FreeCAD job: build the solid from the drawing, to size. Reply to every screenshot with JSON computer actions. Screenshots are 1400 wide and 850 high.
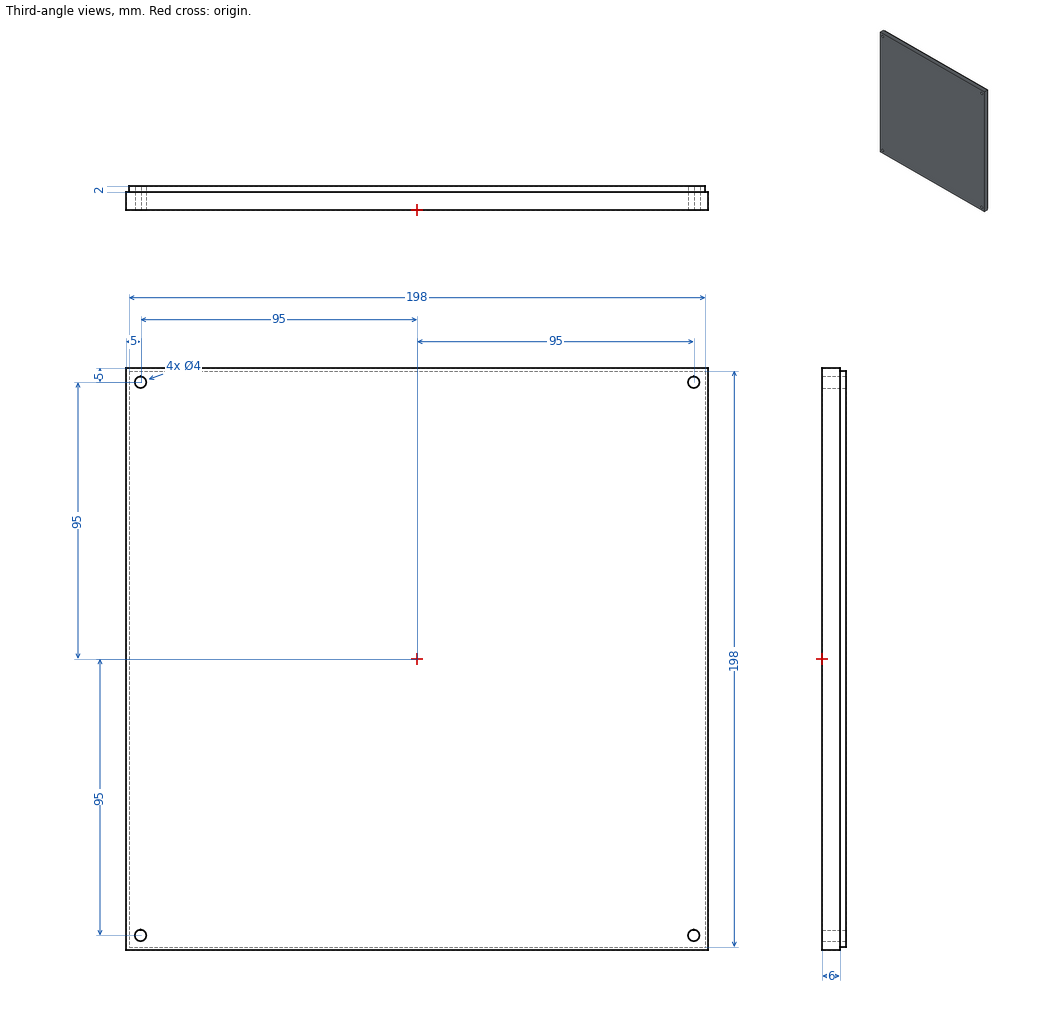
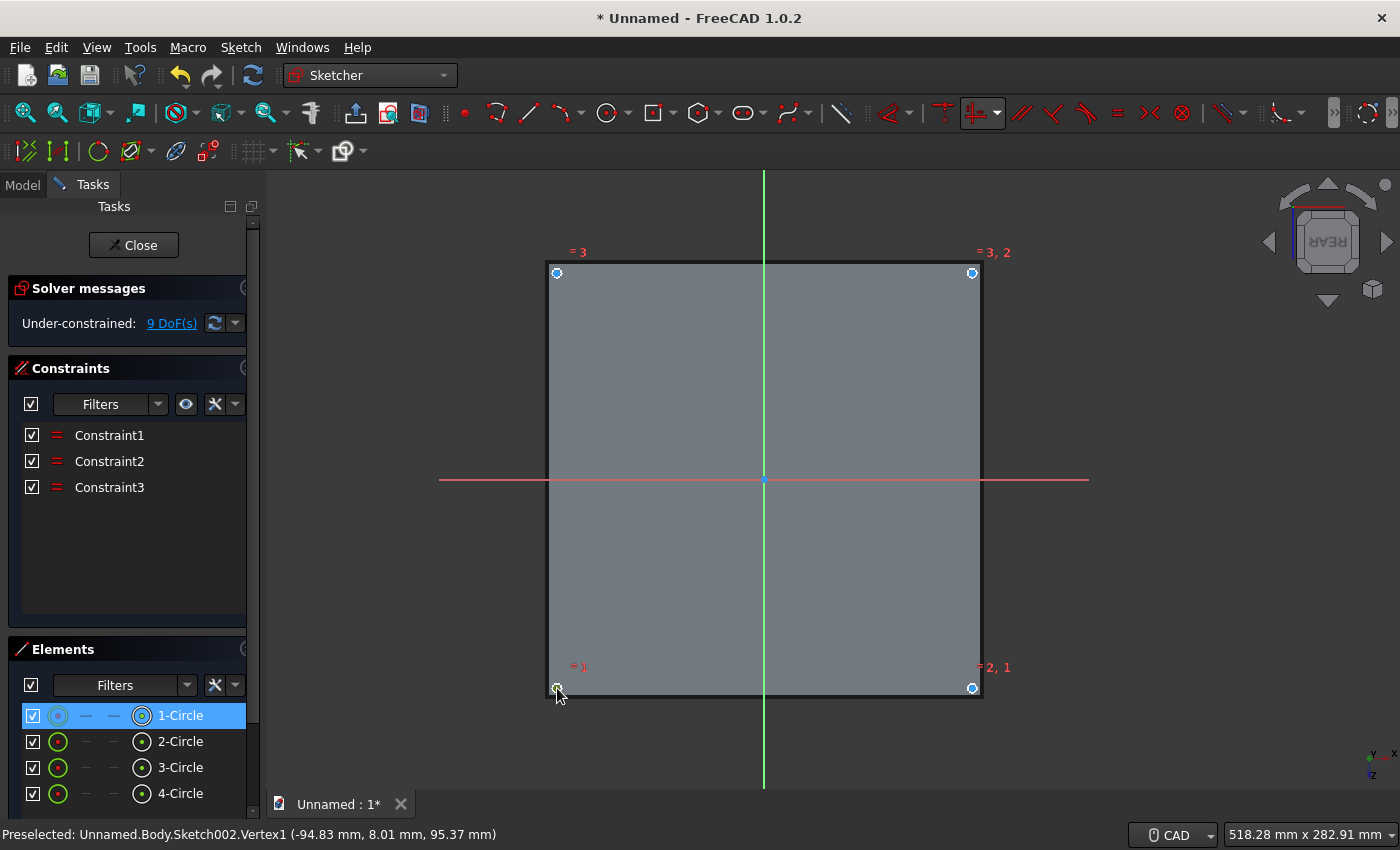
{"action": "left_click", "coordinate": [972, 688]}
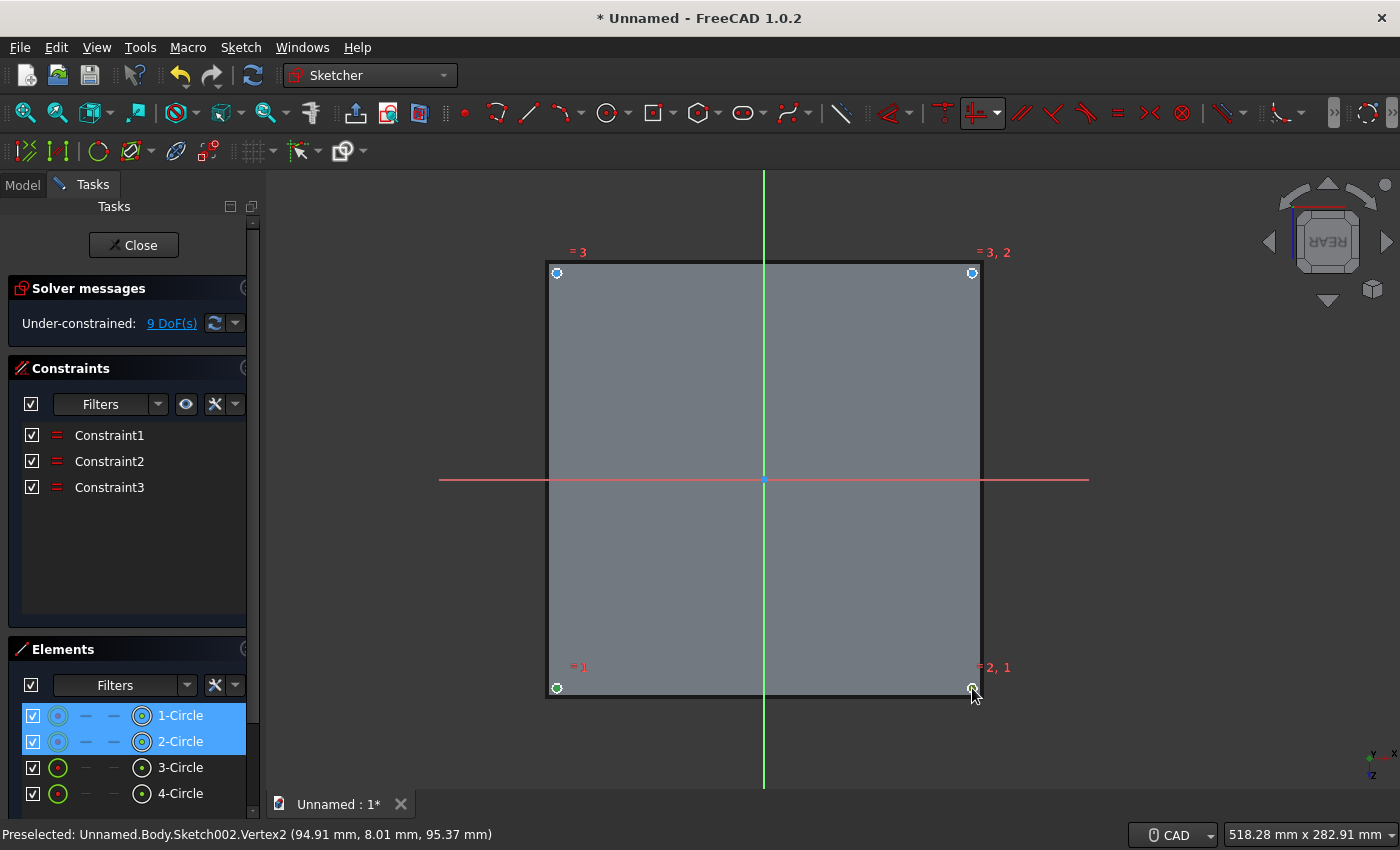
{"action": "left_click", "coordinate": [1000, 114]}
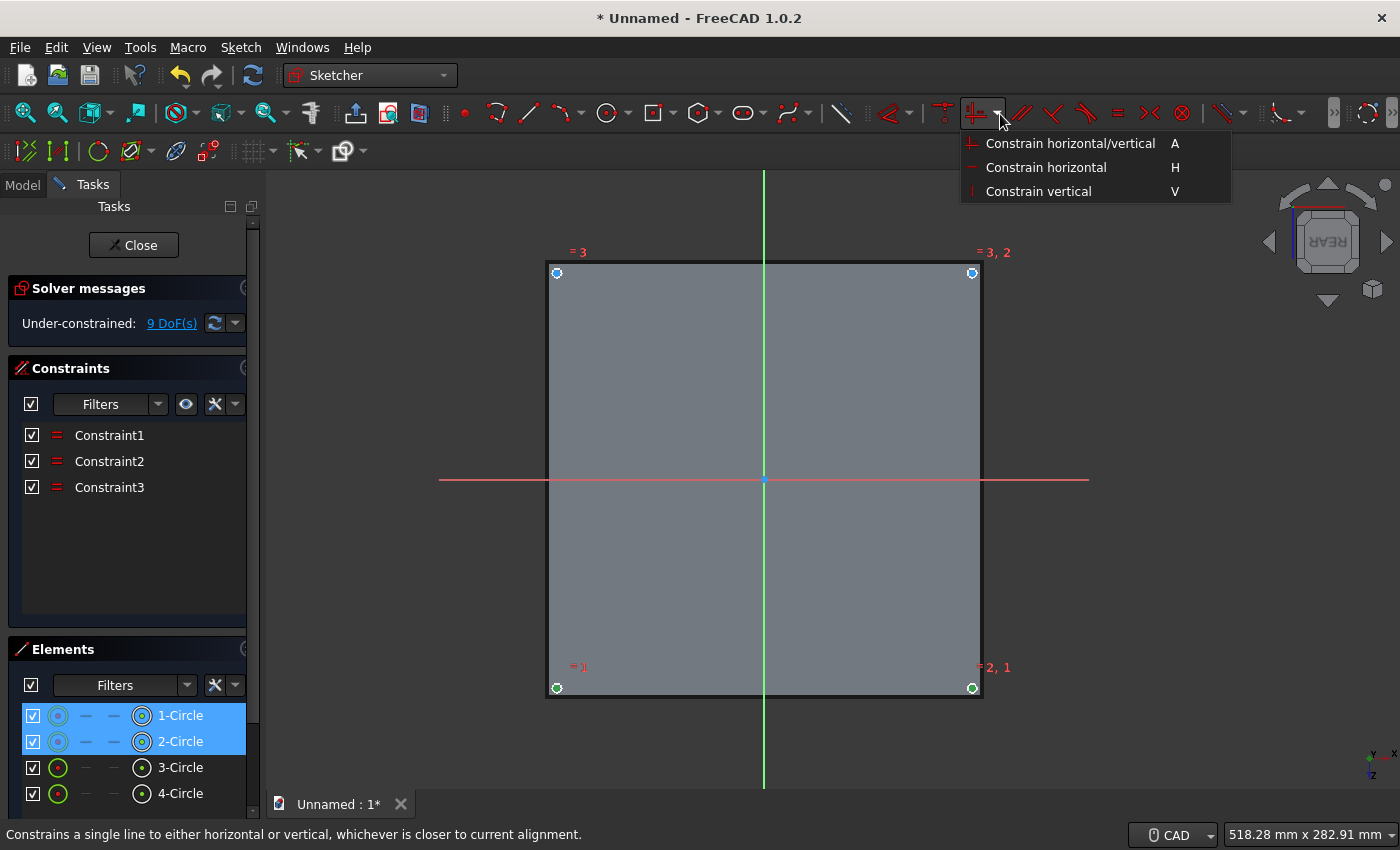
{"action": "left_click", "coordinate": [1096, 167]}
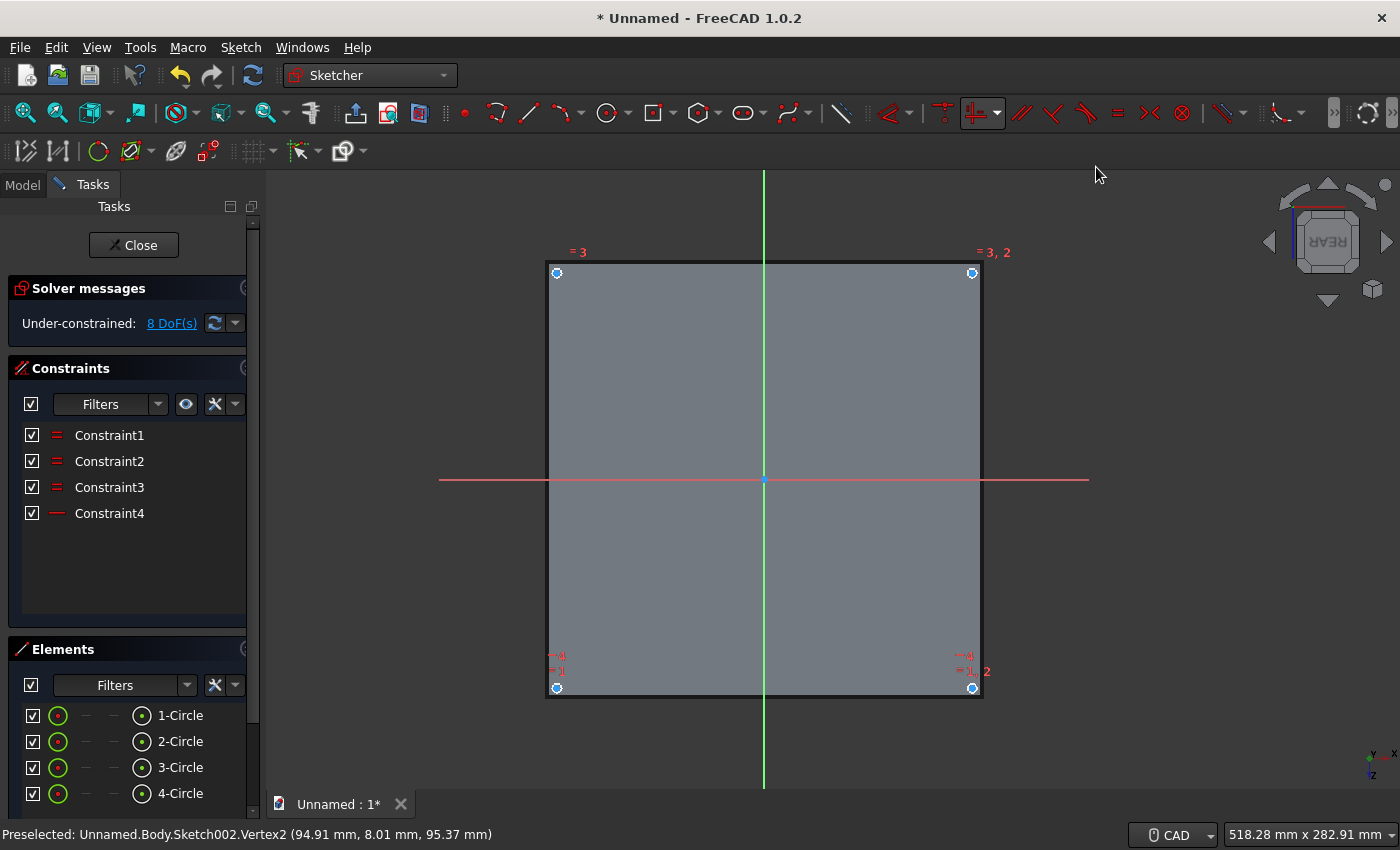
{"action": "left_click", "coordinate": [972, 688]}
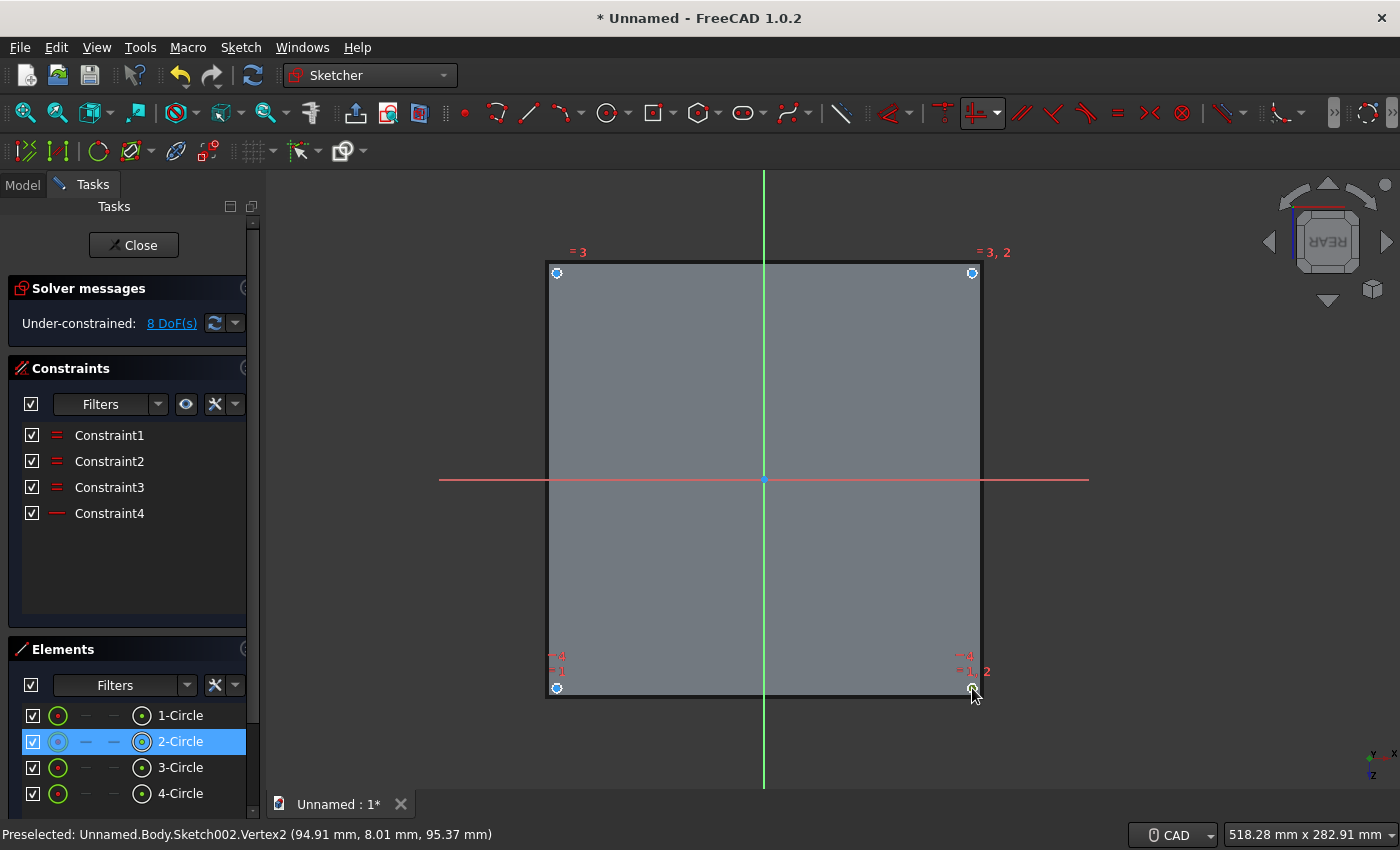
{"action": "left_click", "coordinate": [972, 273]}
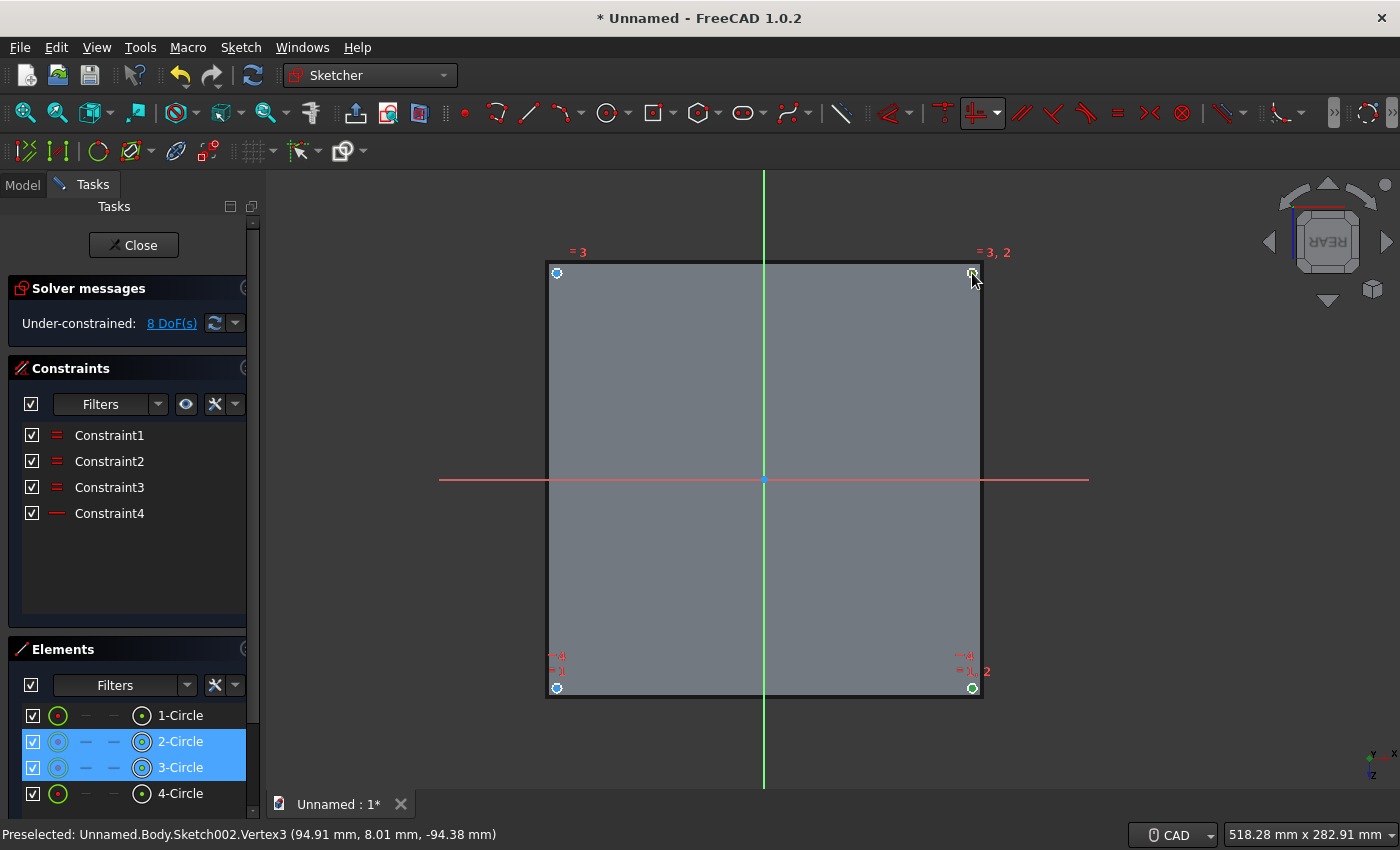
{"action": "key", "text": "v"}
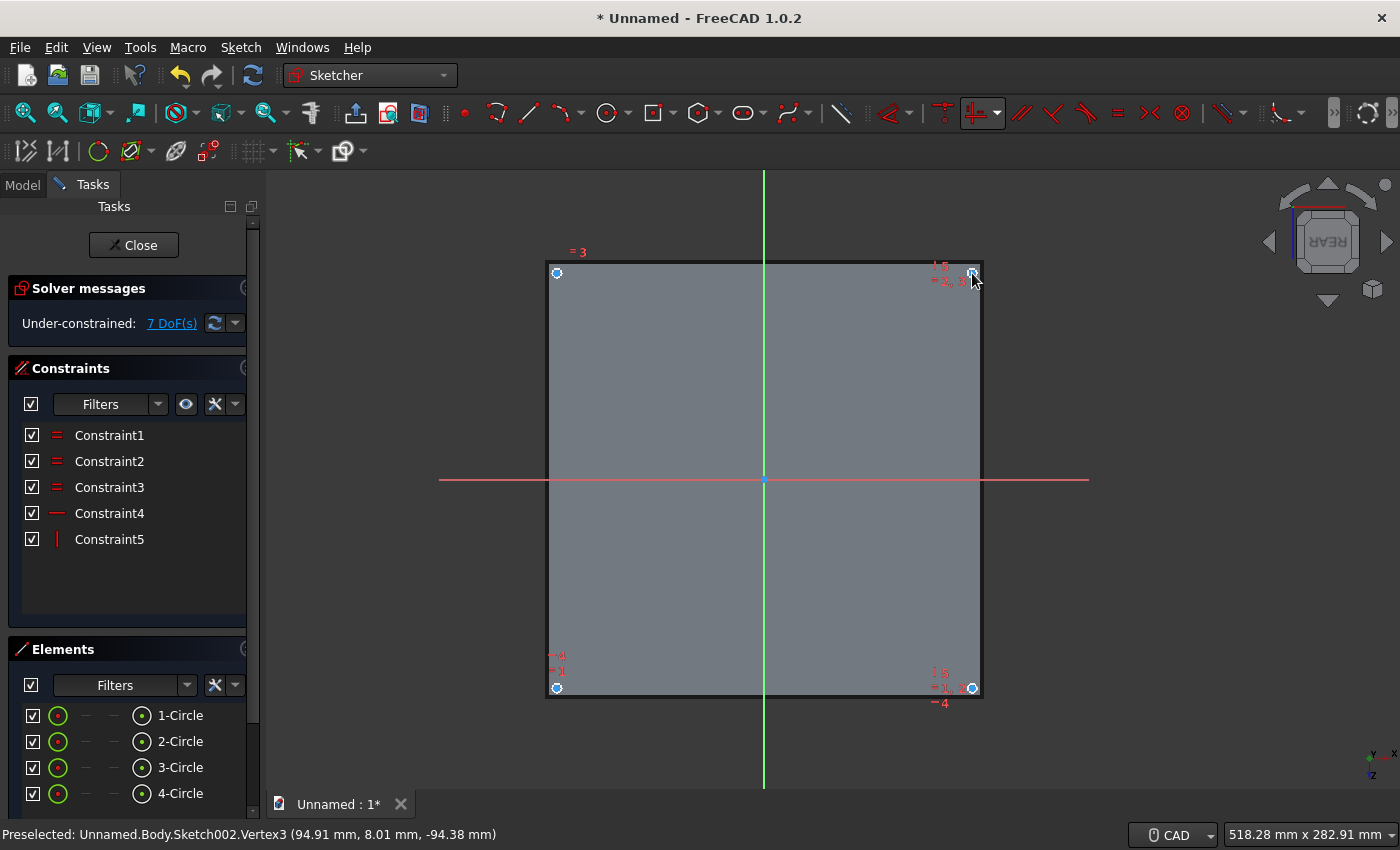
{"action": "left_click", "coordinate": [557, 688]}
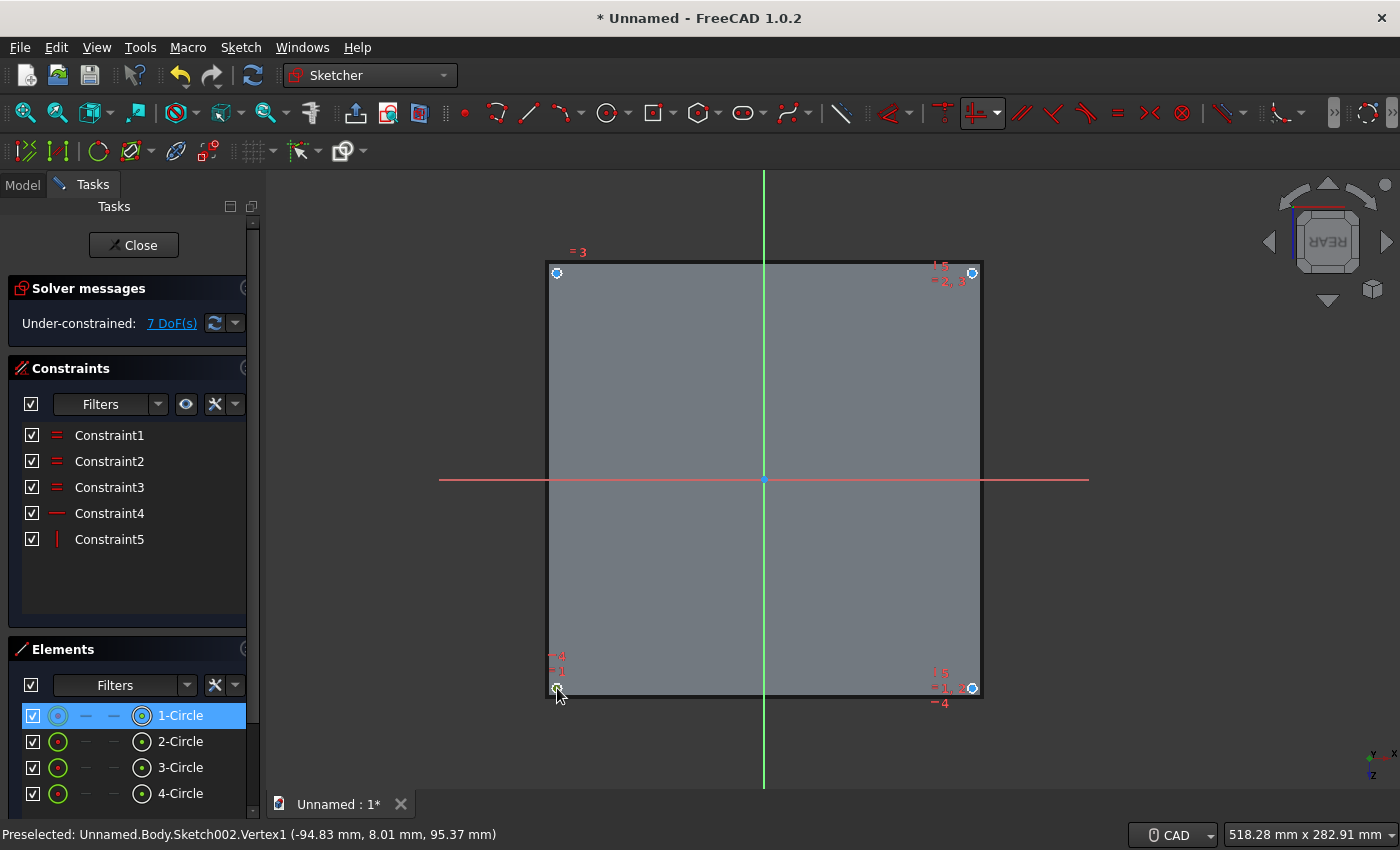
{"action": "left_click", "coordinate": [557, 273]}